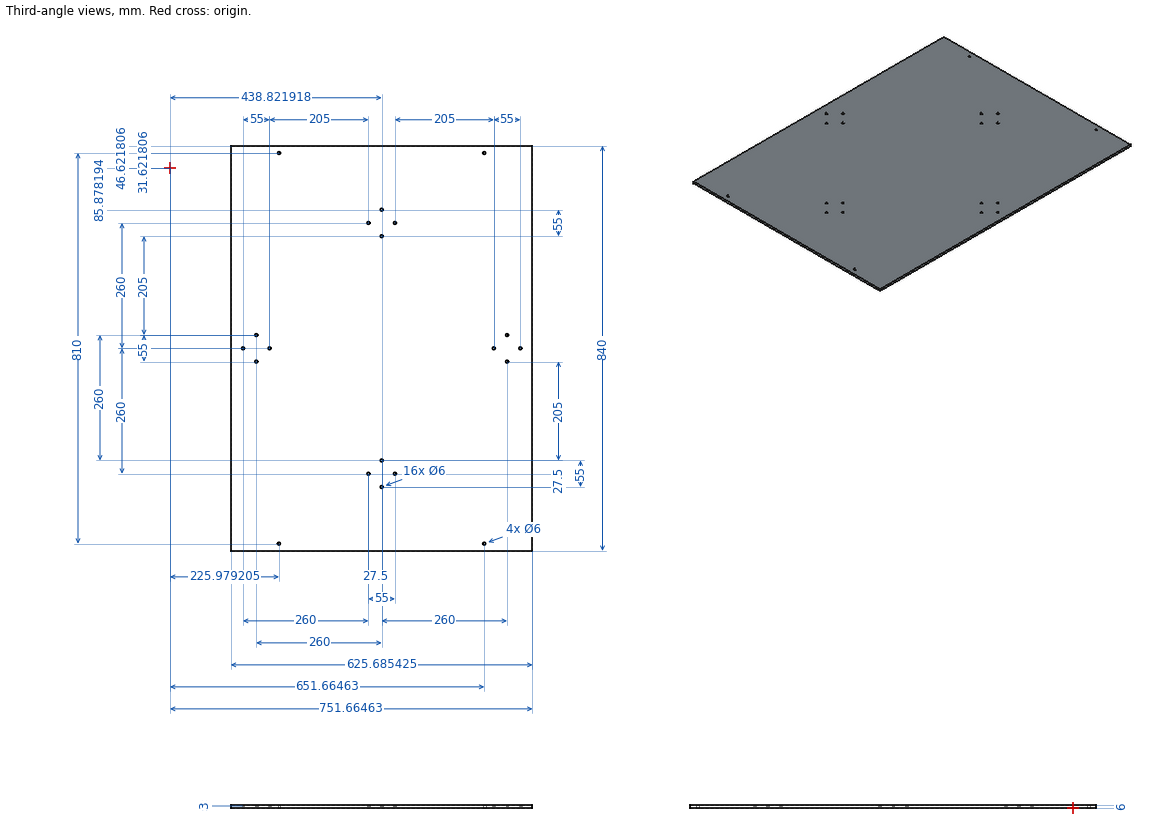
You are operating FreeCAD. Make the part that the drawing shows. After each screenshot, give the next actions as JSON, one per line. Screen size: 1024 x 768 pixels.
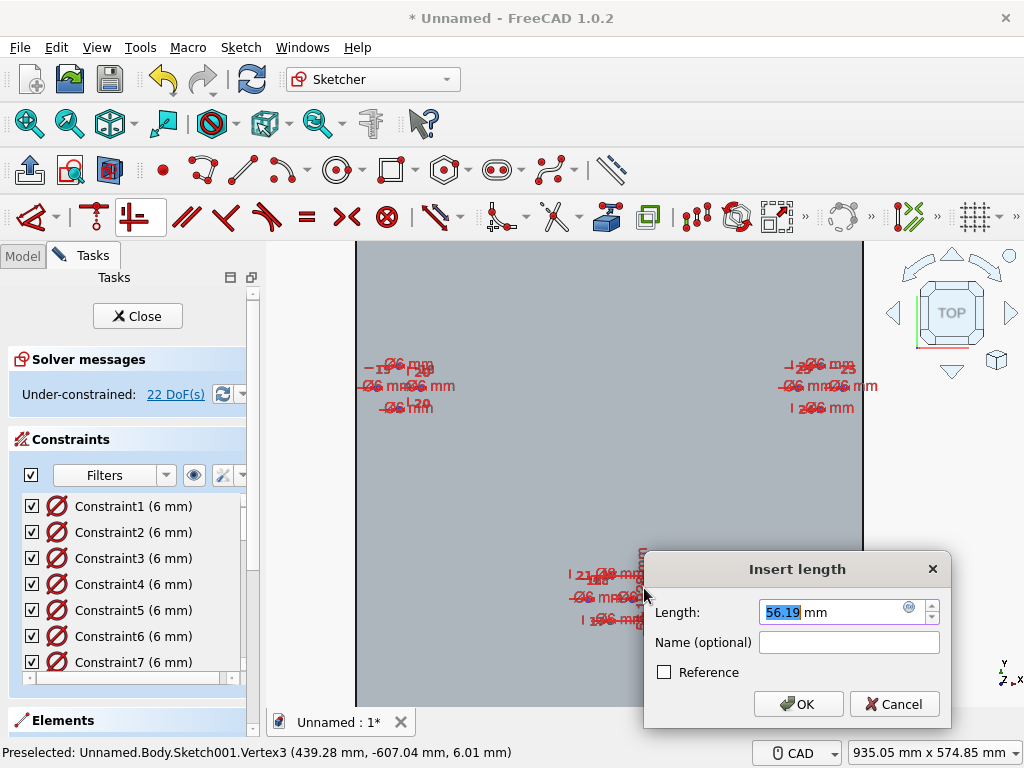
{"action": "type", "text": "55"}
{"action": "key", "text": "Return"}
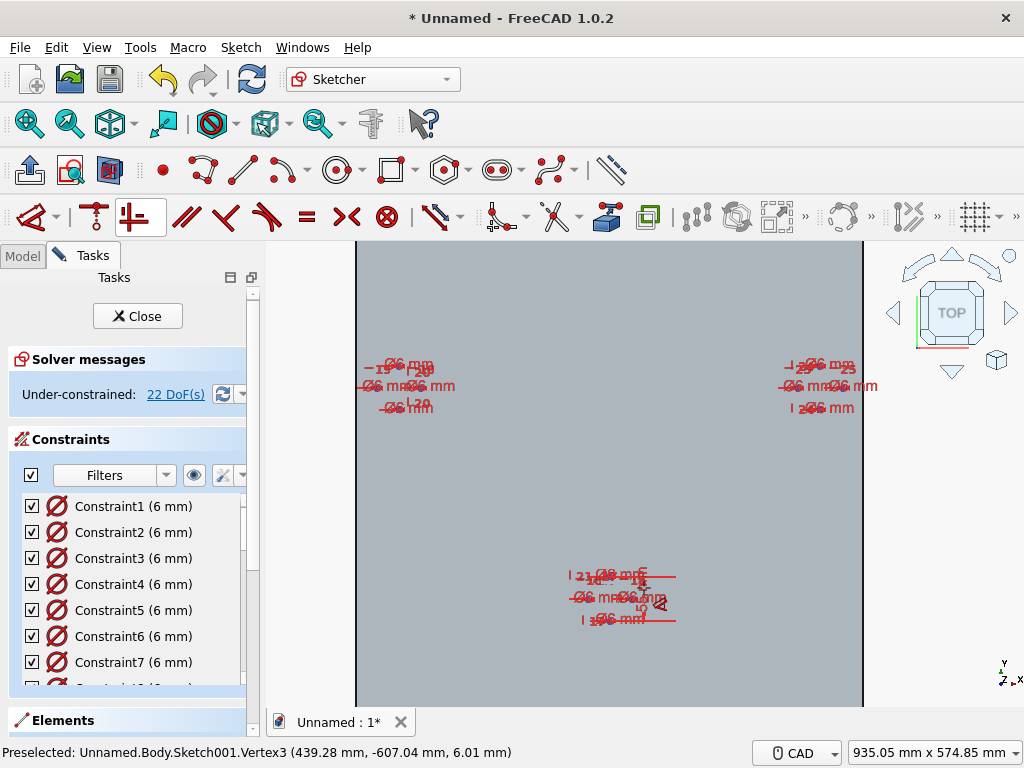
{"action": "left_click", "coordinate": [588, 599]}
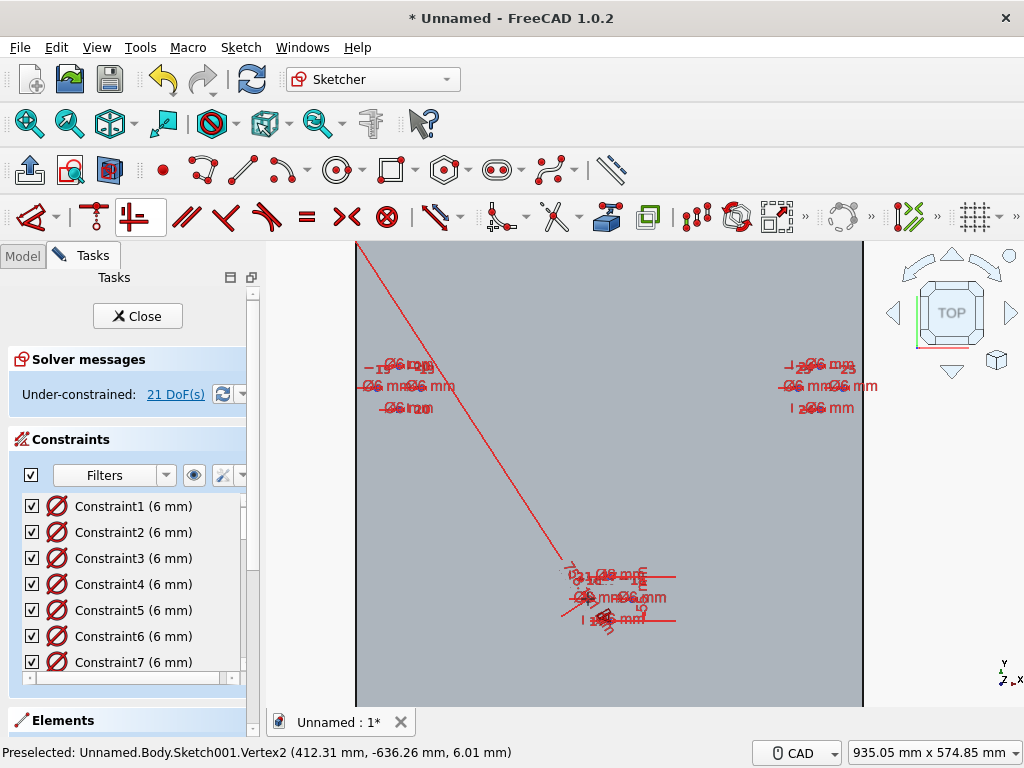
{"action": "left_click", "coordinate": [631, 599]}
{"action": "left_click", "coordinate": [600, 633]}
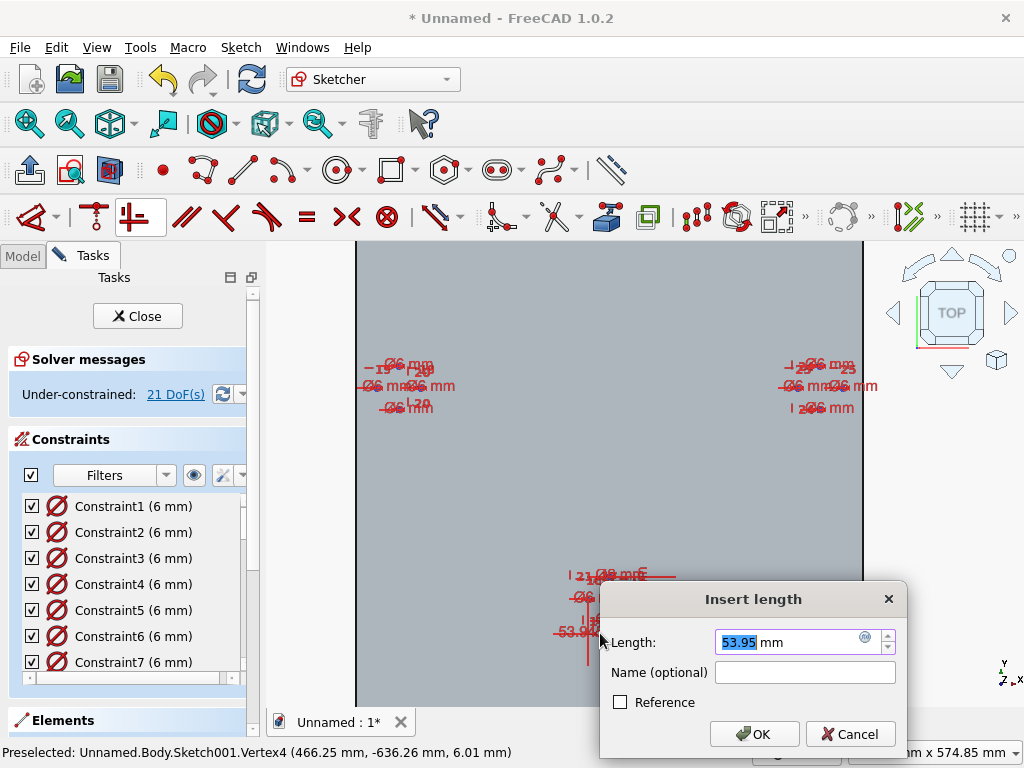
{"action": "type", "text": "55"}
{"action": "key", "text": "Return"}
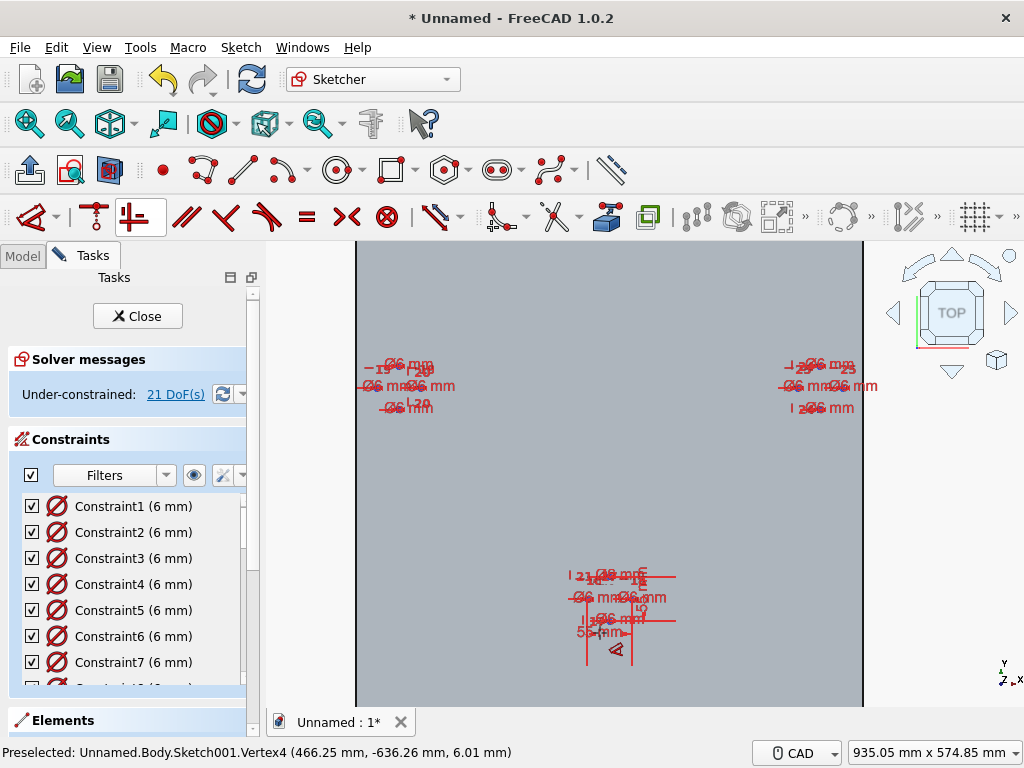
{"action": "left_click", "coordinate": [376, 388]}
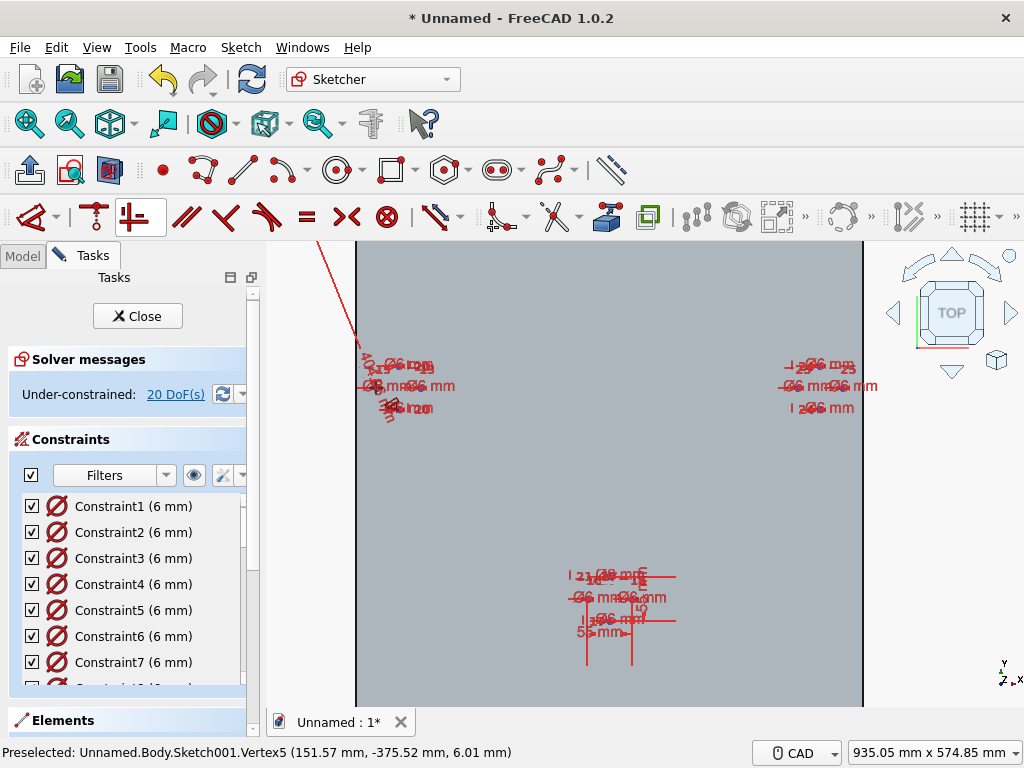
{"action": "left_click", "coordinate": [420, 388]}
{"action": "left_click", "coordinate": [388, 422]}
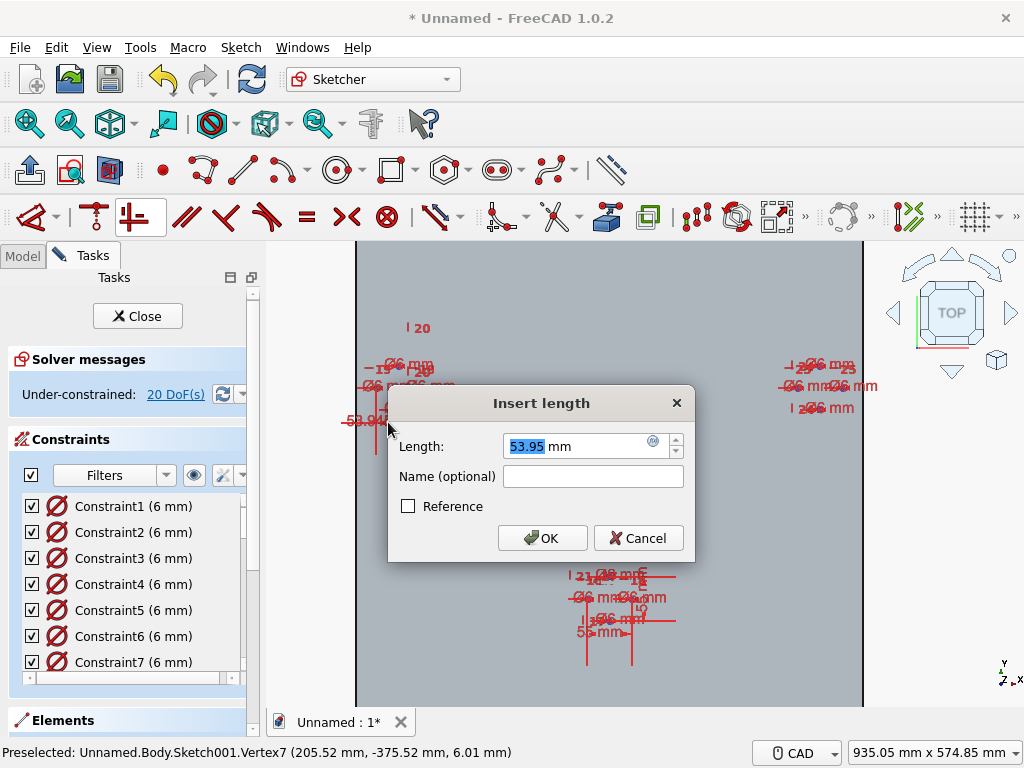
{"action": "type", "text": "55"}
{"action": "key", "text": "Return"}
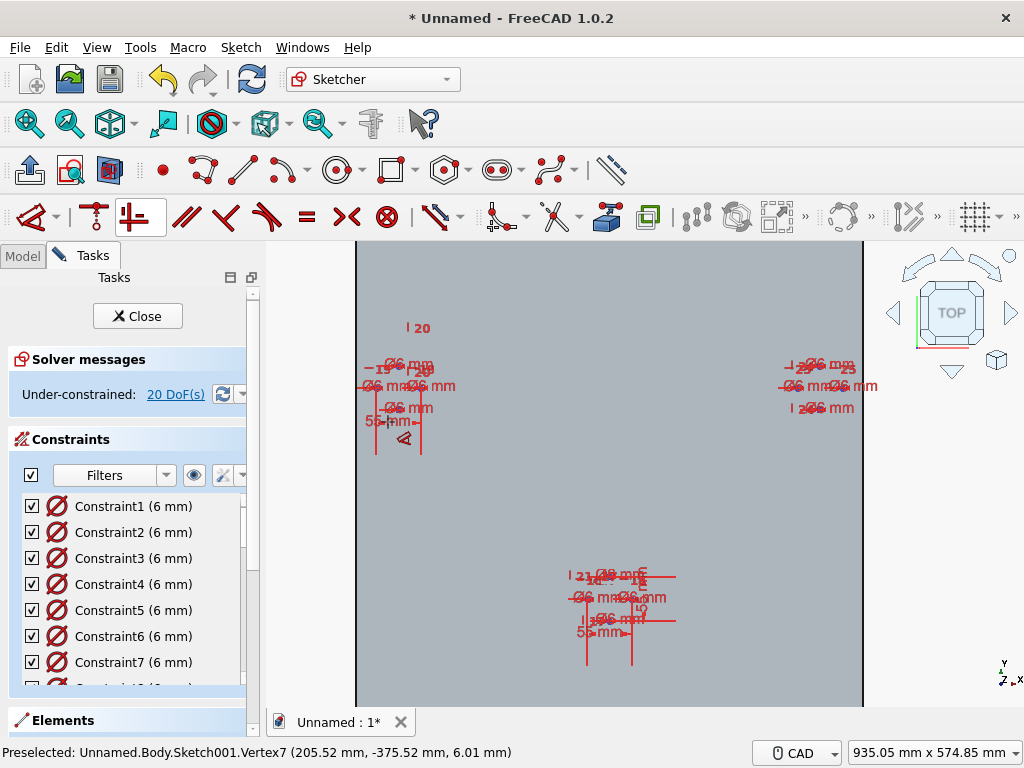
{"action": "left_click", "coordinate": [398, 366]}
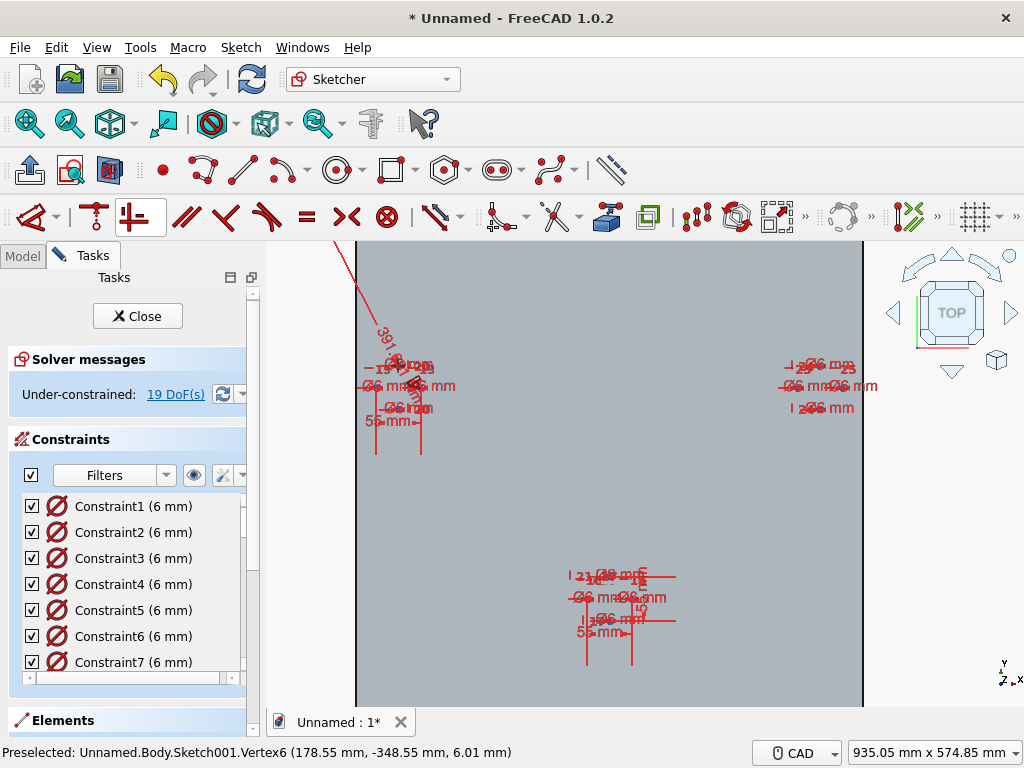
{"action": "left_click", "coordinate": [398, 410]}
{"action": "left_click", "coordinate": [364, 378]}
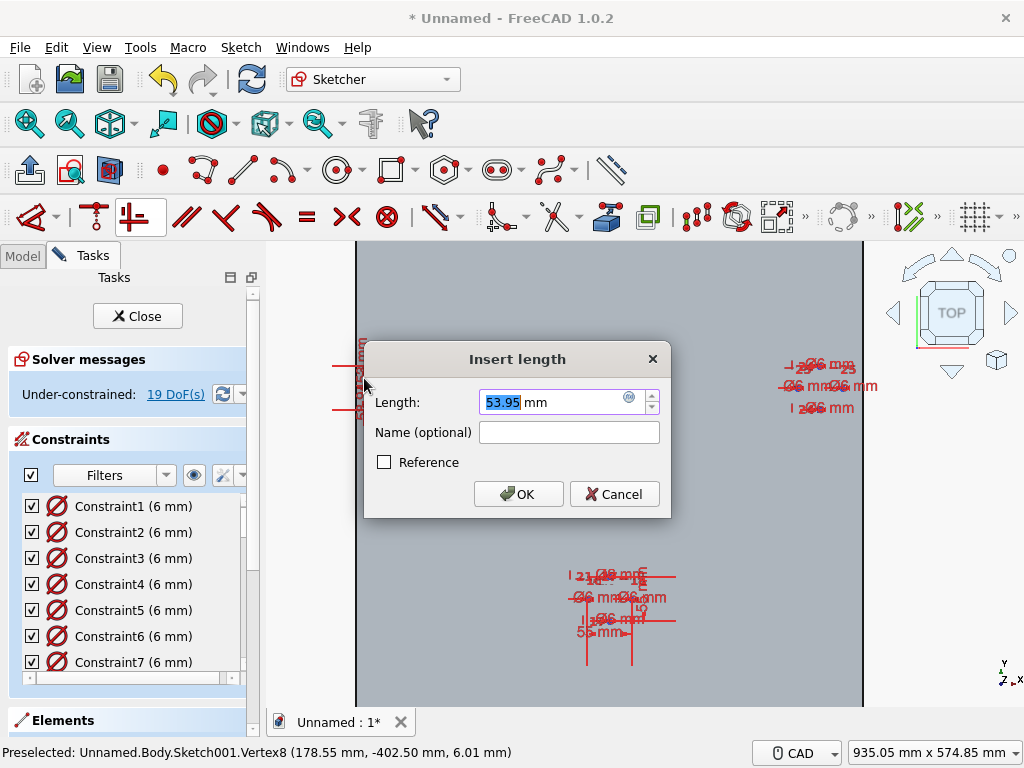
{"action": "type", "text": "55"}
{"action": "key", "text": "Return"}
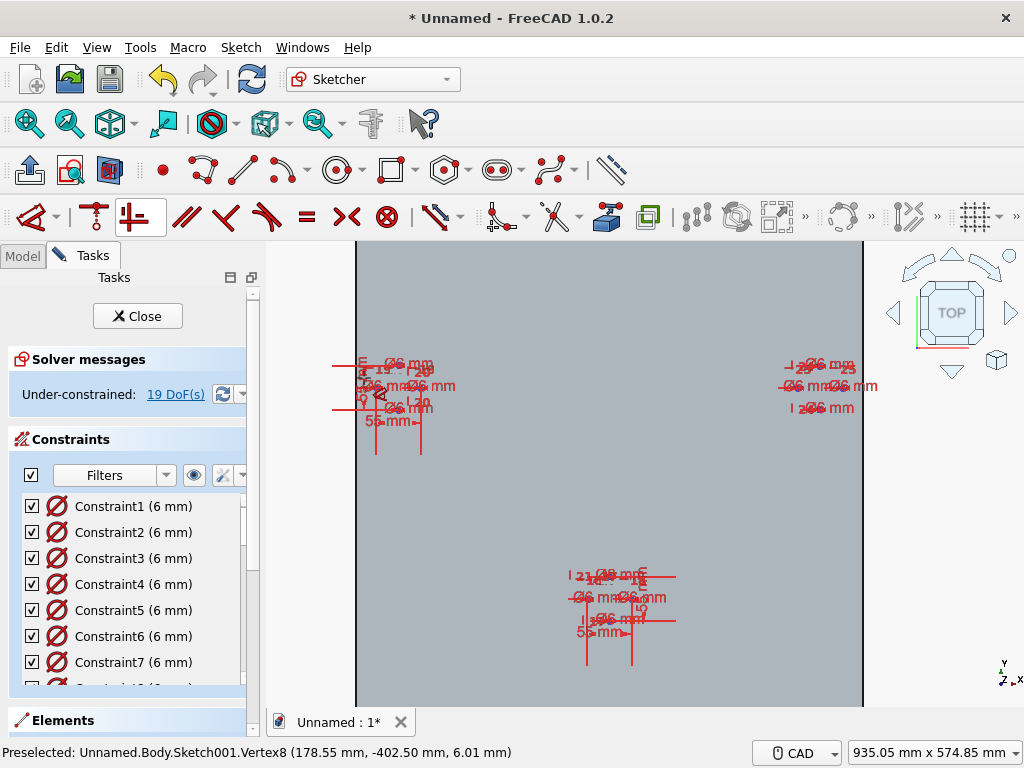
{"action": "scroll", "coordinate": [610, 621], "scroll_direction": "down", "scroll_amount": 3}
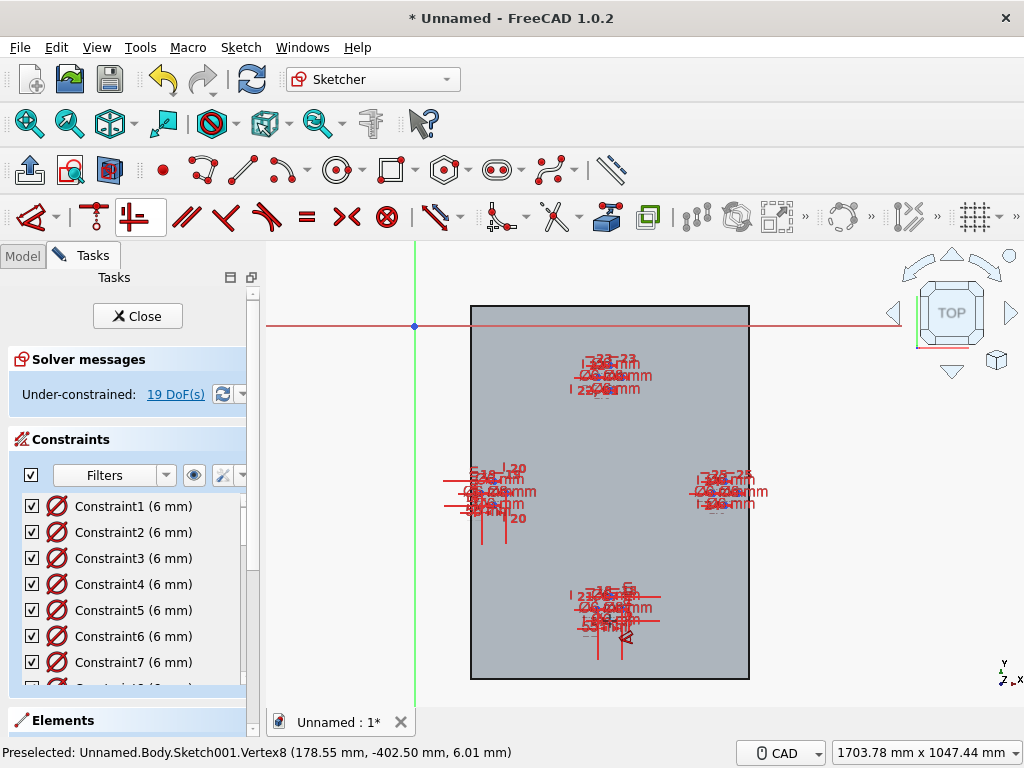
{"action": "scroll", "coordinate": [610, 391], "scroll_direction": "up", "scroll_amount": 3}